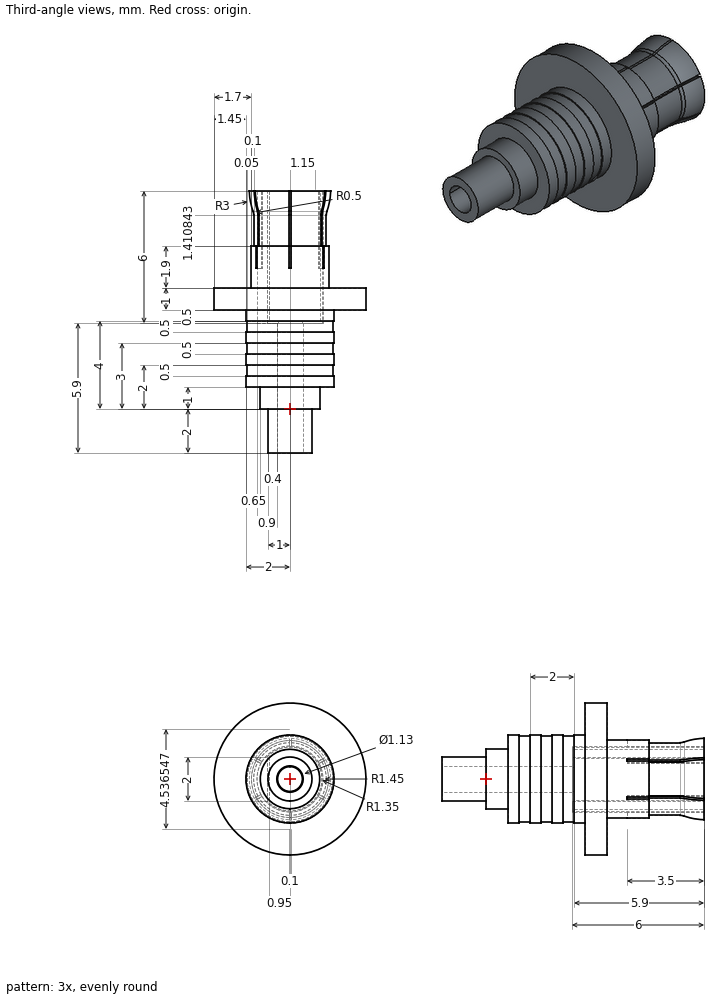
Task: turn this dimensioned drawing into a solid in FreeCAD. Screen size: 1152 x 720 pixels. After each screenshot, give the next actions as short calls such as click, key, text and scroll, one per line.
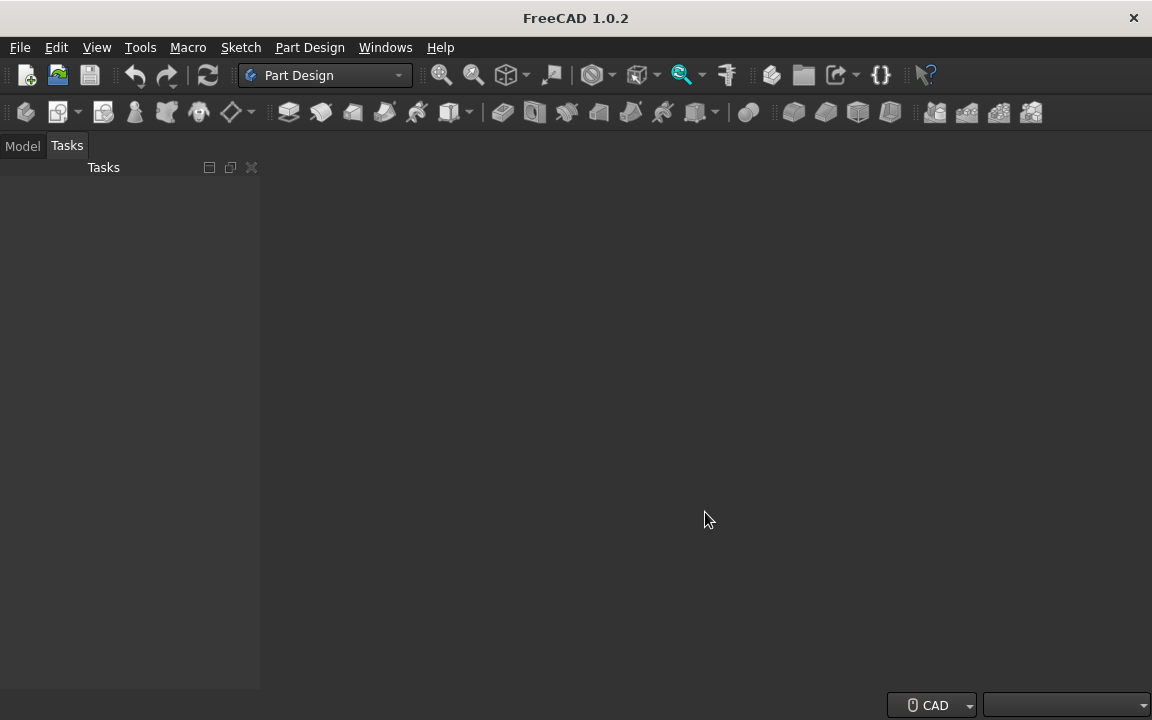
click(26, 76)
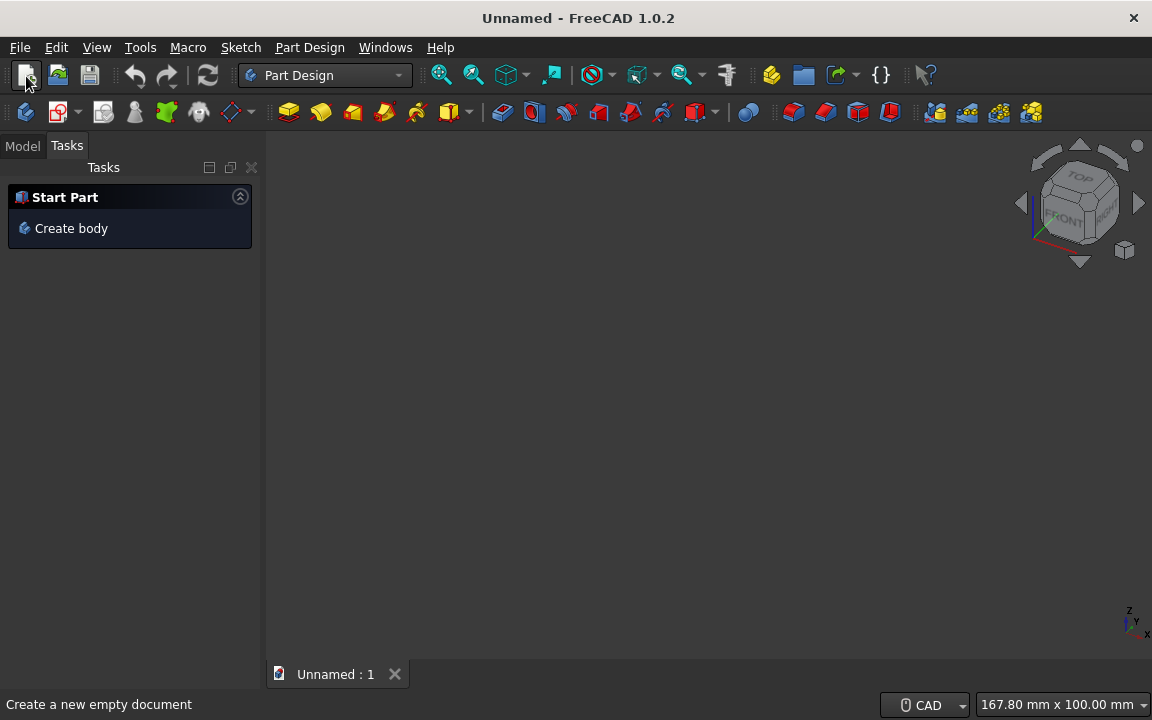
click(58, 112)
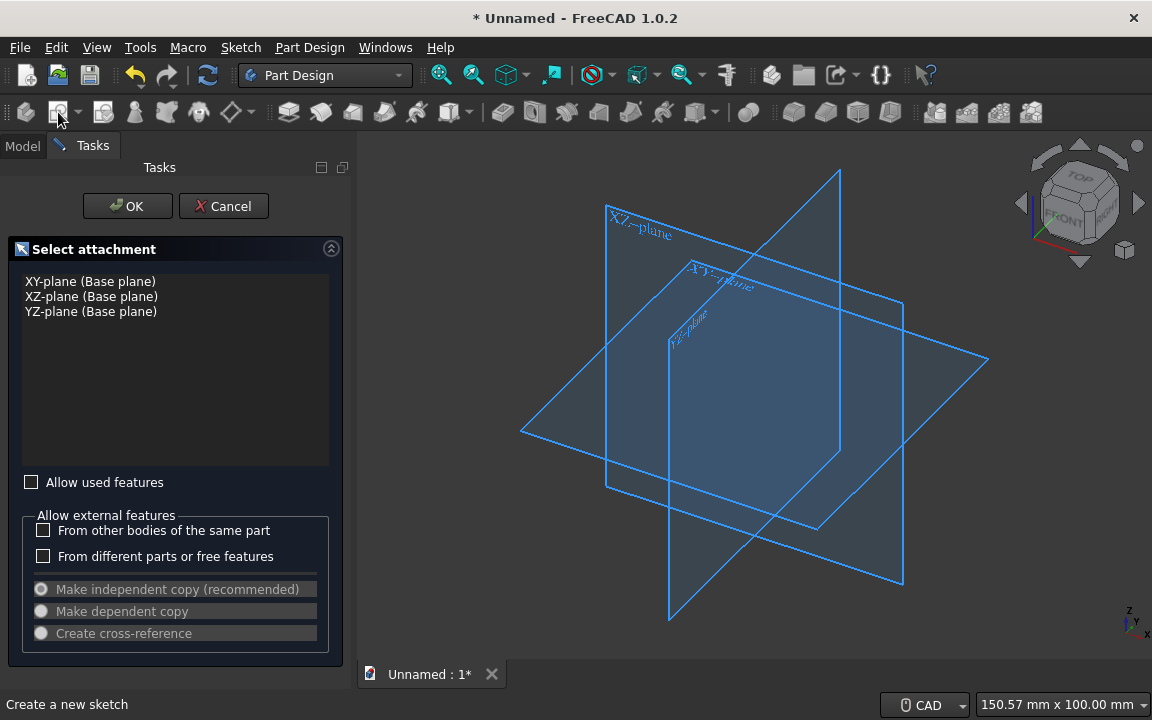
click(82, 282)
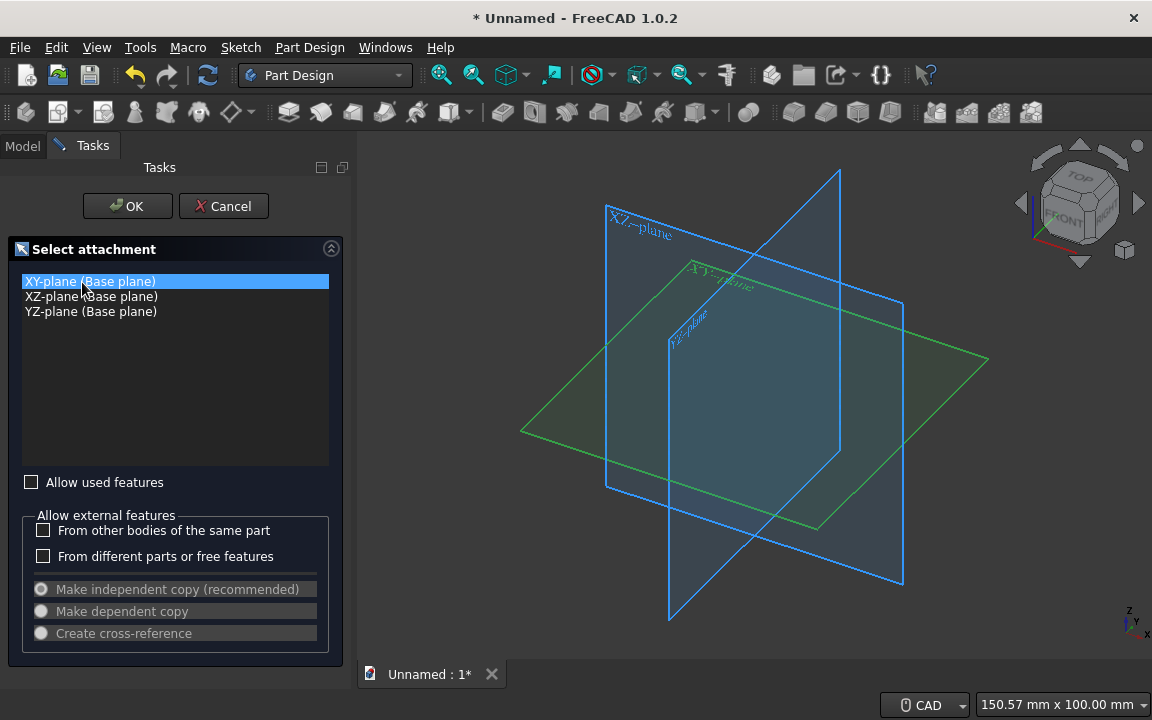
click(128, 206)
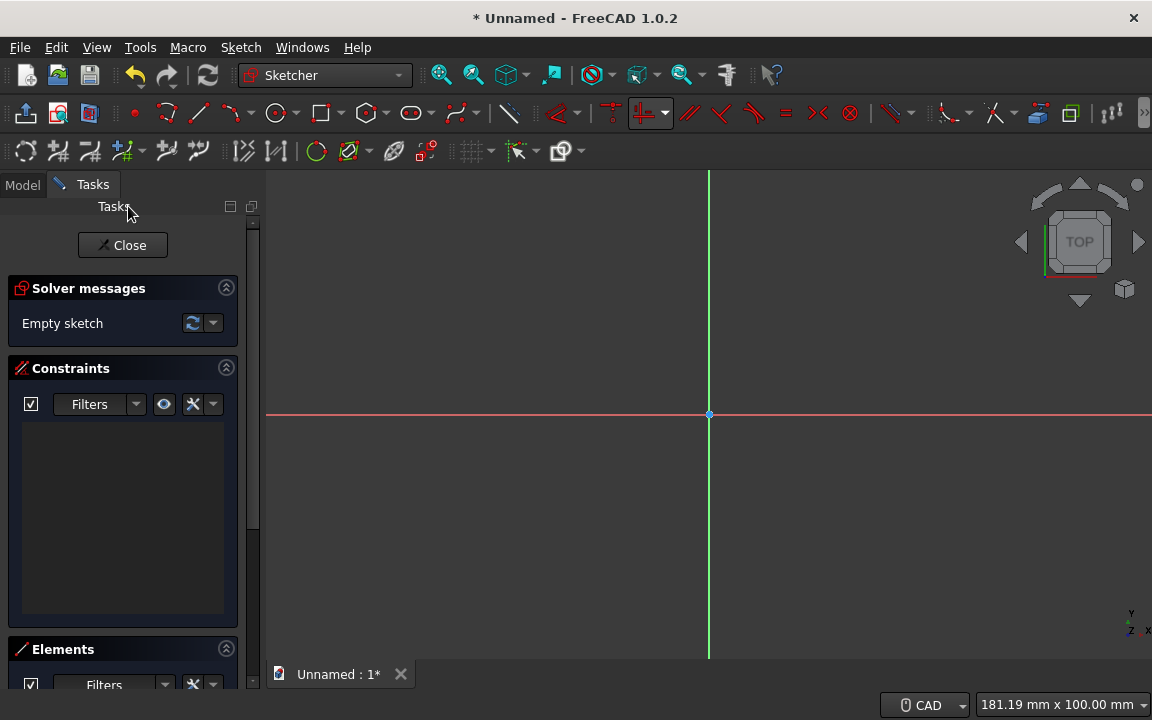
scroll(716, 390, up, 8)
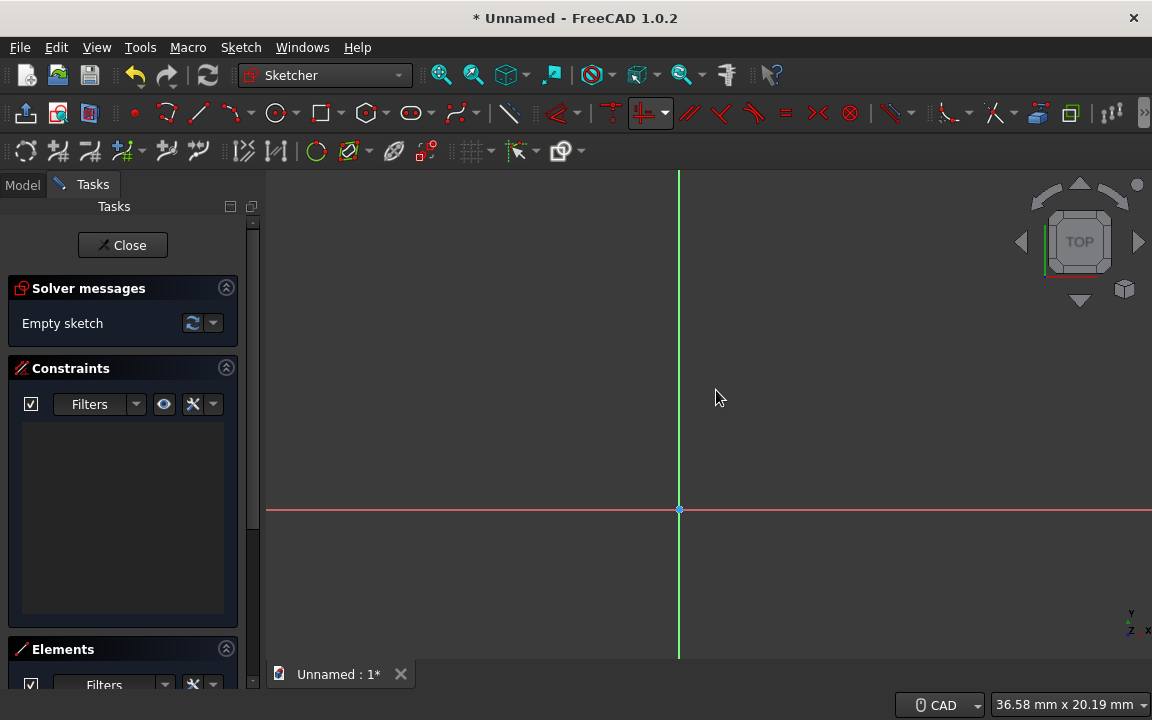
click(168, 114)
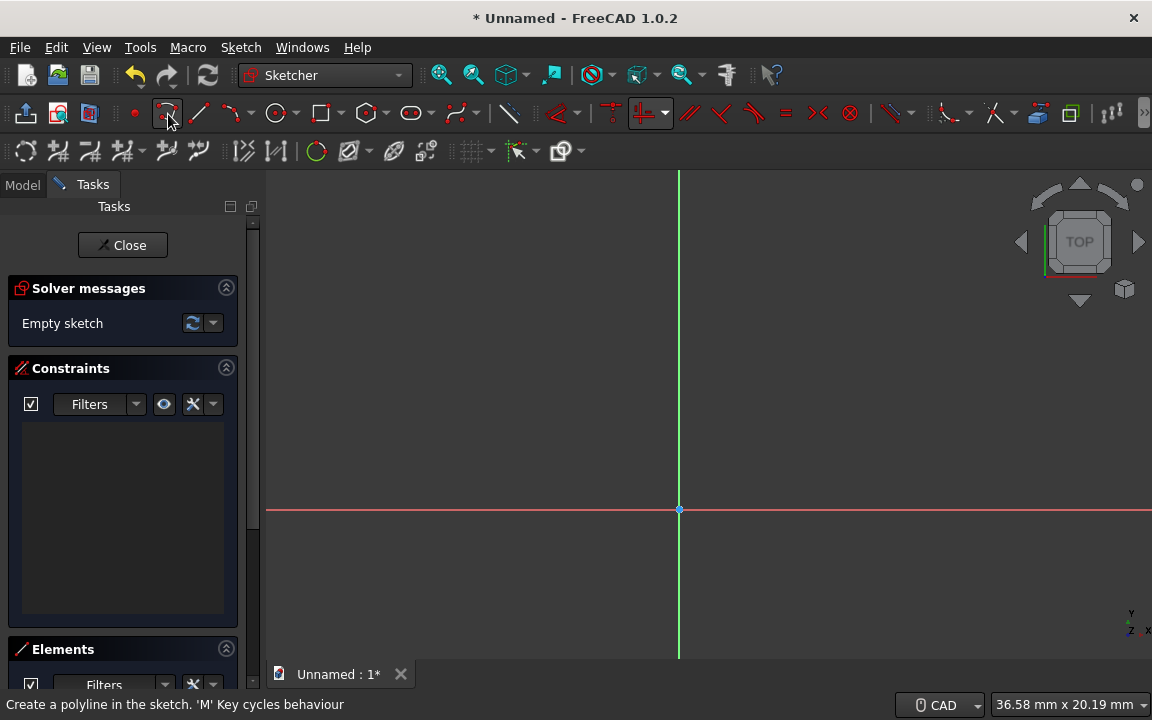
click(639, 296)
click(639, 330)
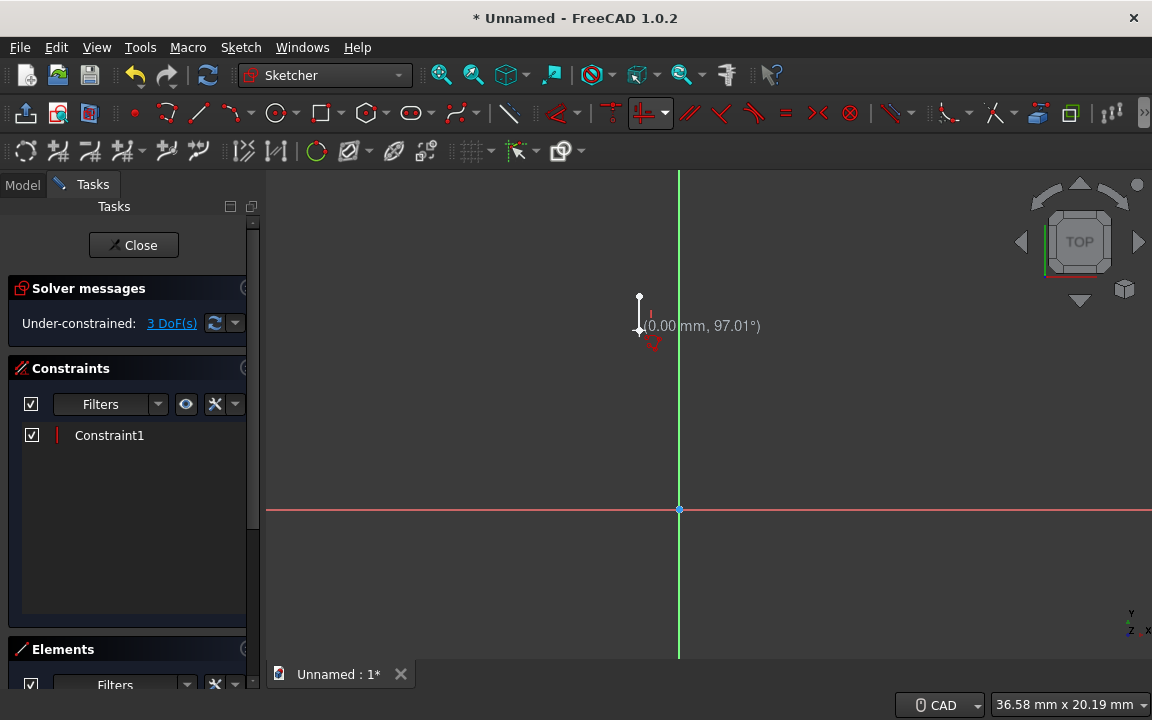
scroll(637, 330, up, 10)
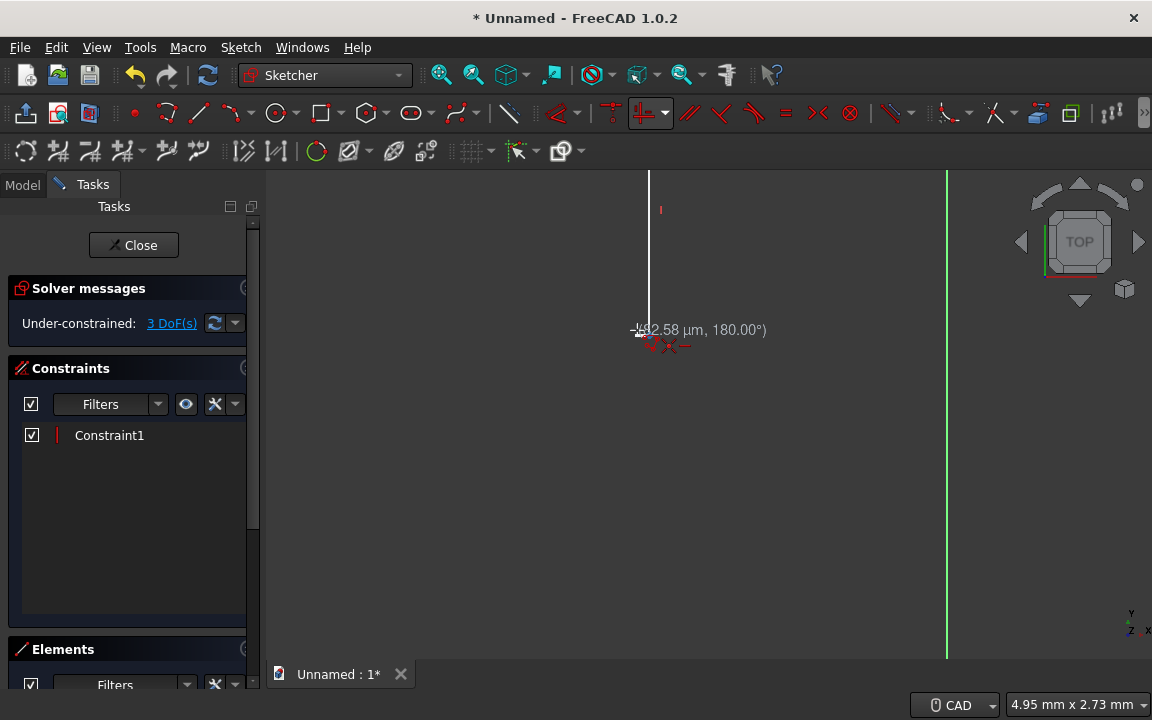
click(634, 328)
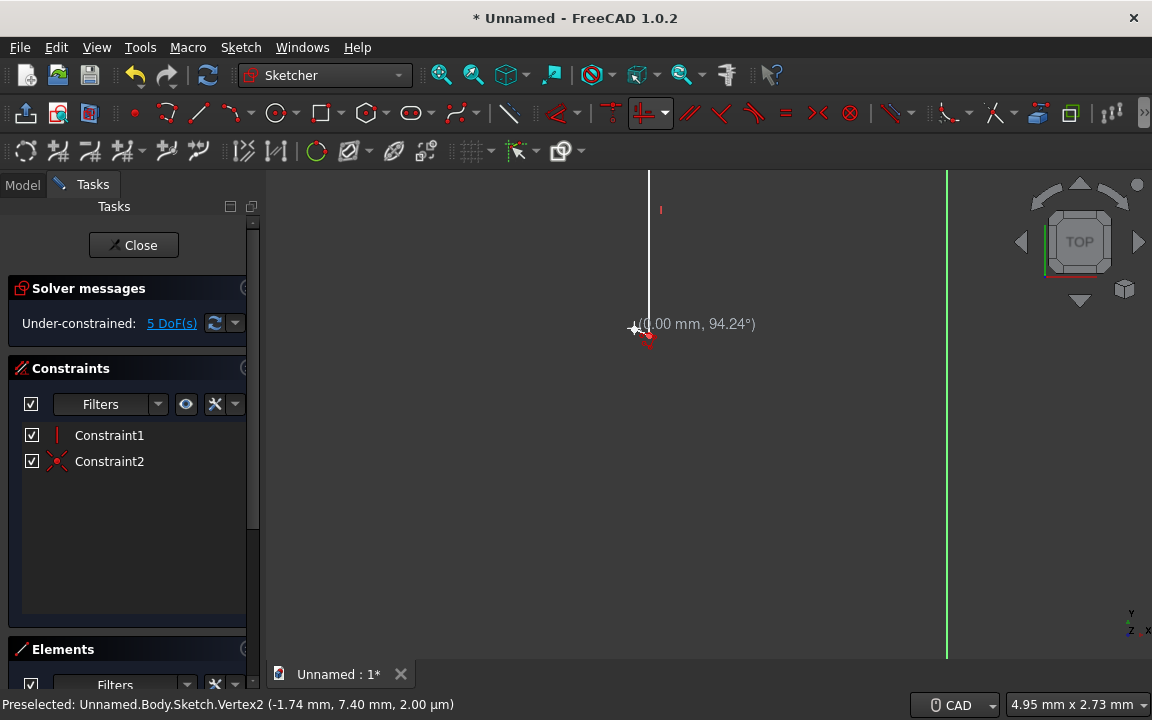
scroll(641, 331, down, 10)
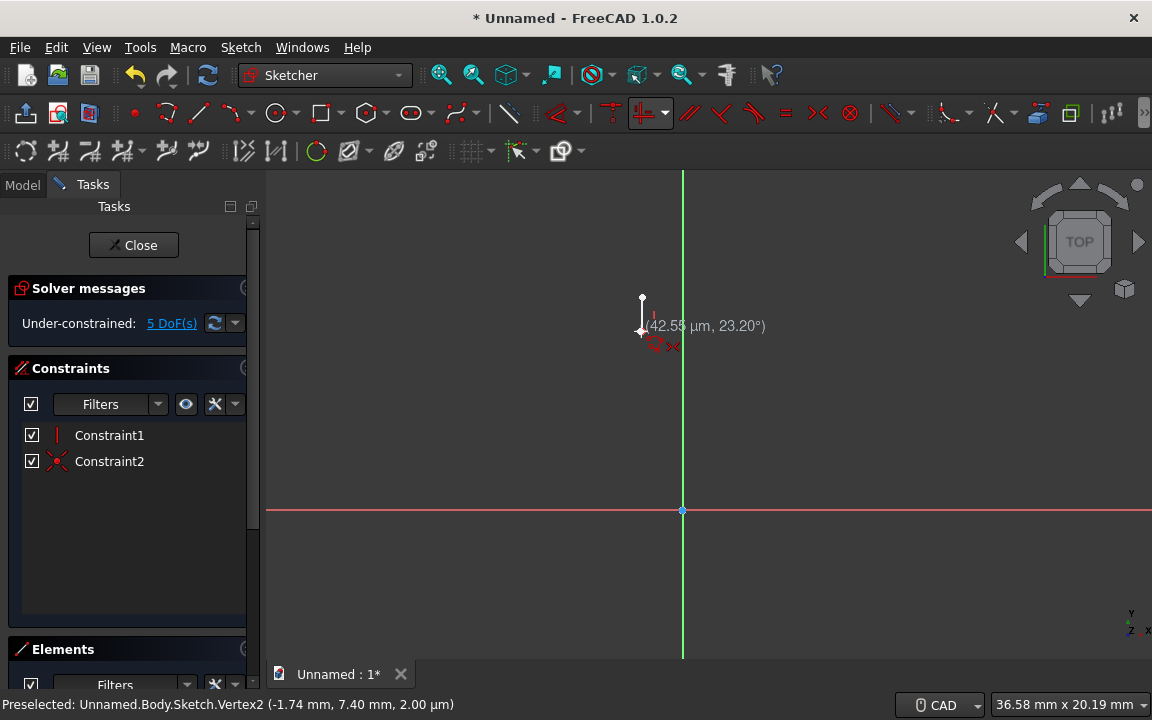
click(640, 377)
click(599, 377)
click(599, 401)
click(634, 401)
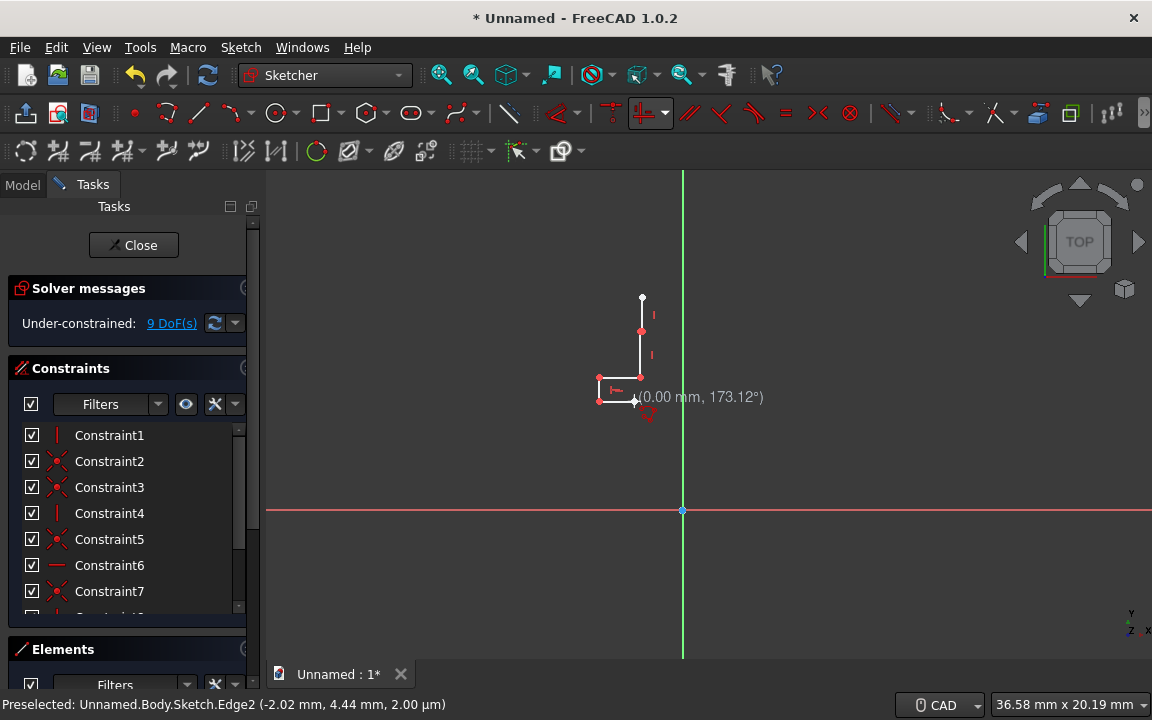
scroll(634, 414, up, 2)